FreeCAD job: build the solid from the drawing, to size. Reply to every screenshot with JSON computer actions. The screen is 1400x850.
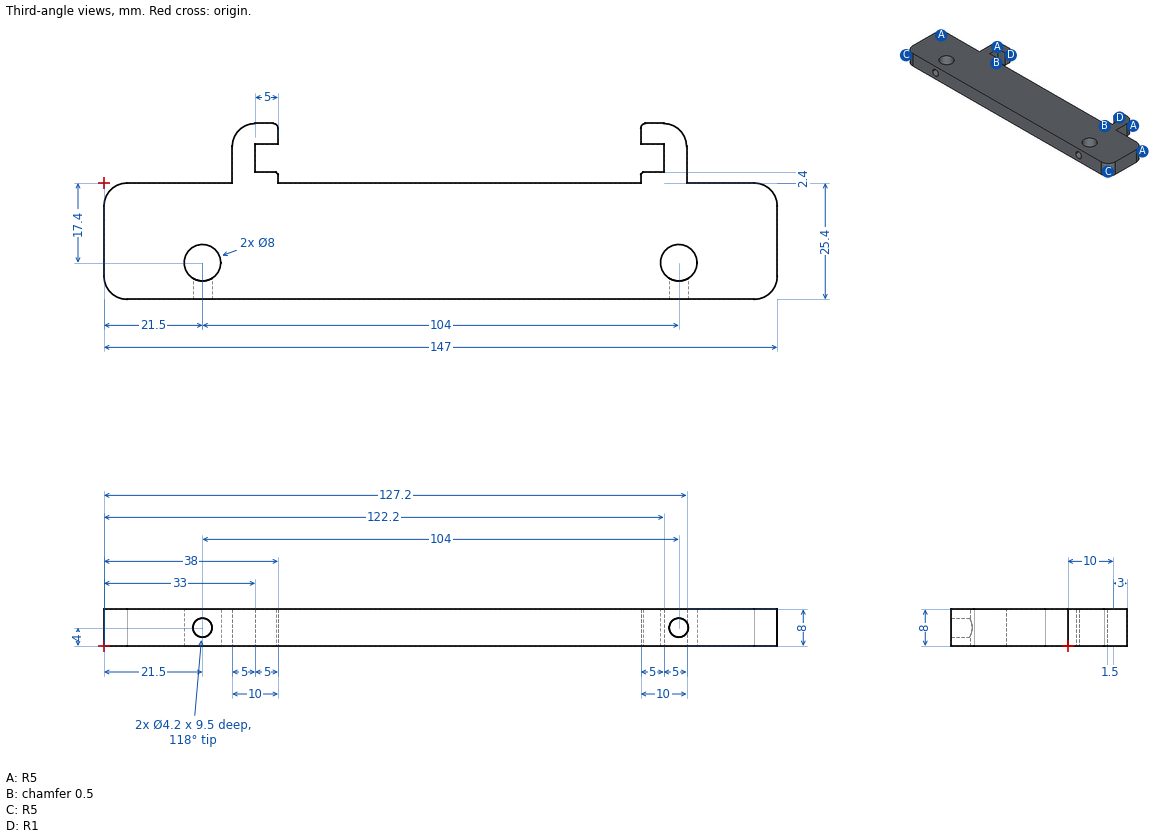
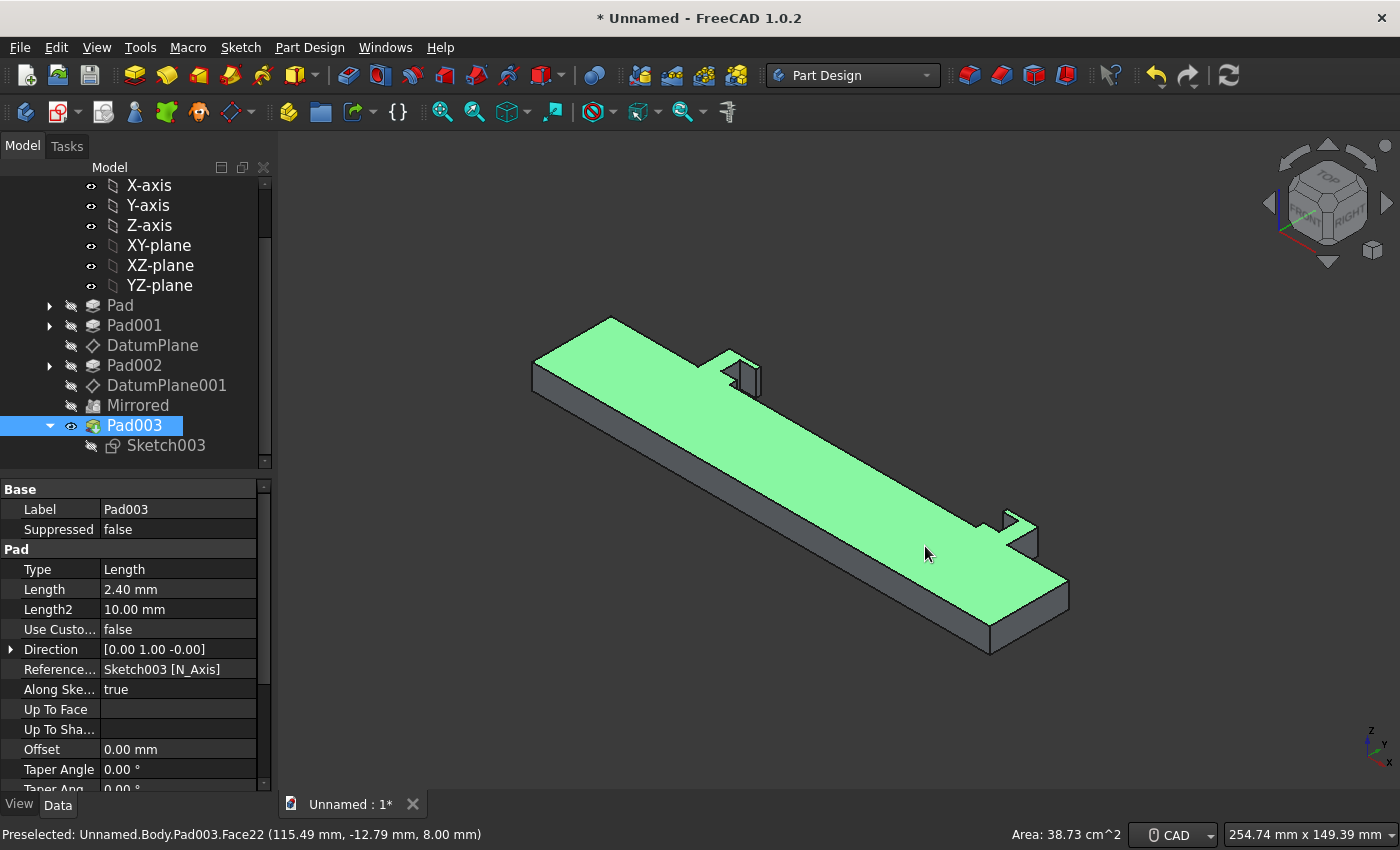
{"action": "left_click", "coordinate": [58, 112]}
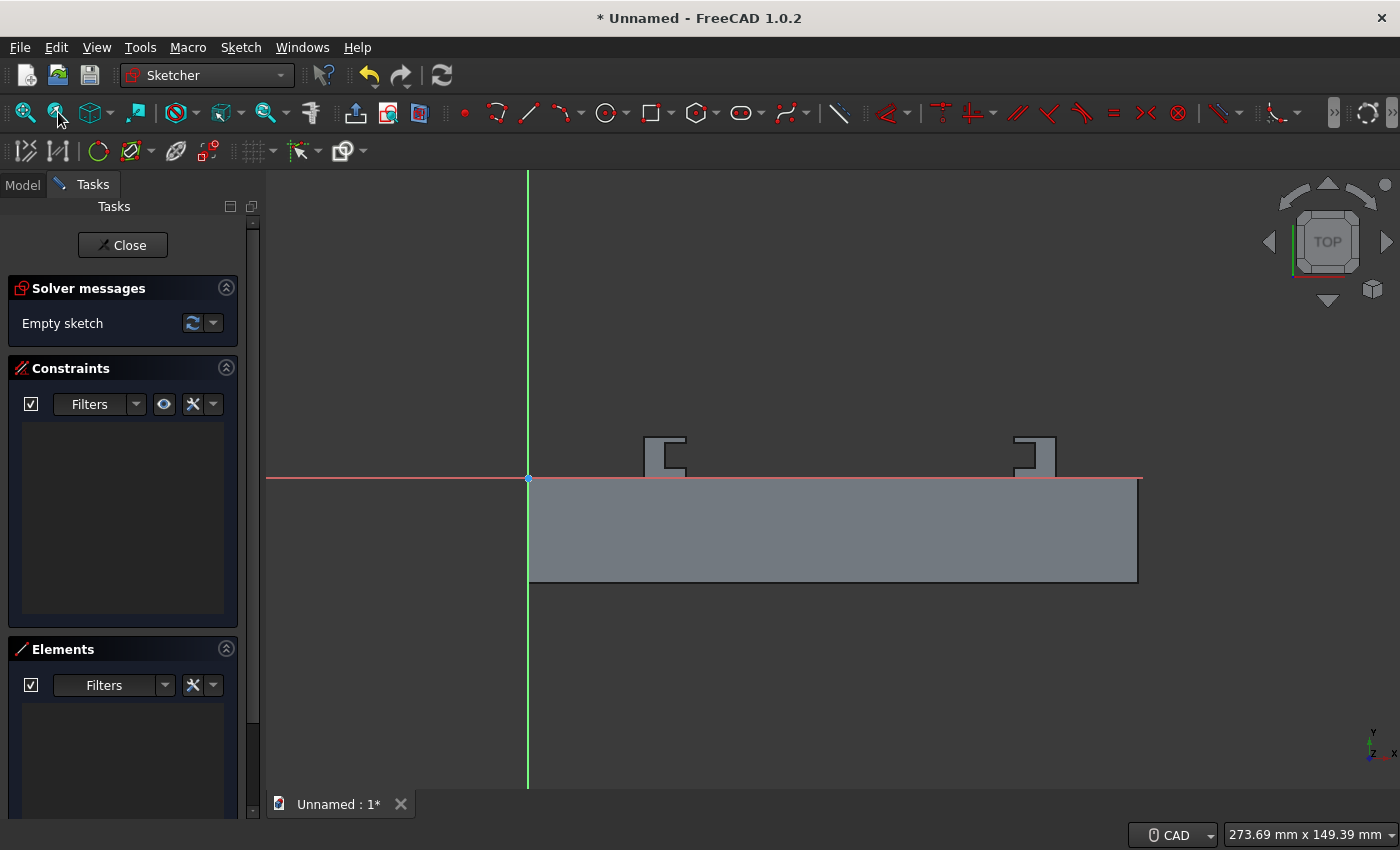
{"action": "left_click", "coordinate": [606, 114]}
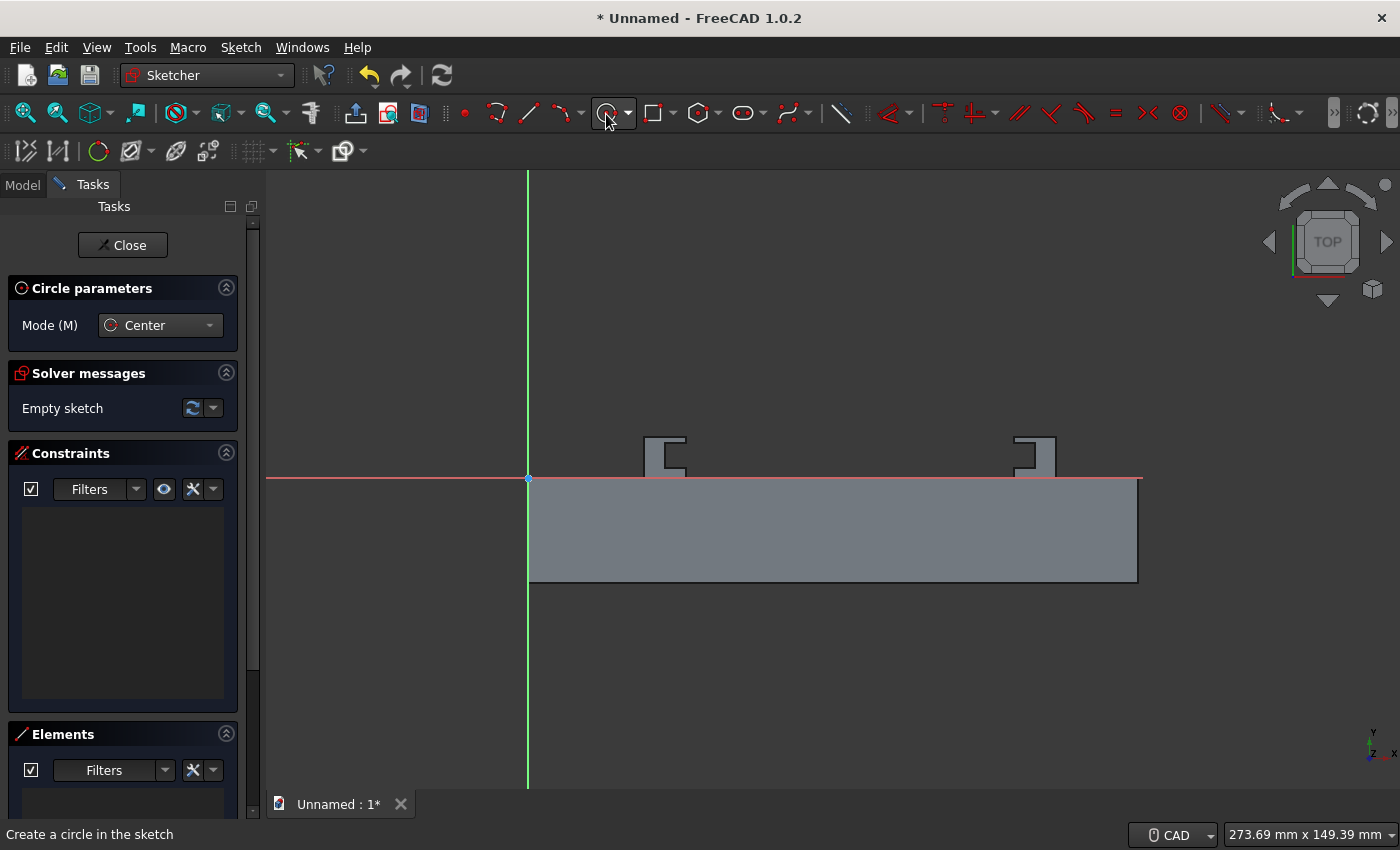
{"action": "scroll", "coordinate": [618, 550], "scroll_direction": "up", "scroll_amount": 2}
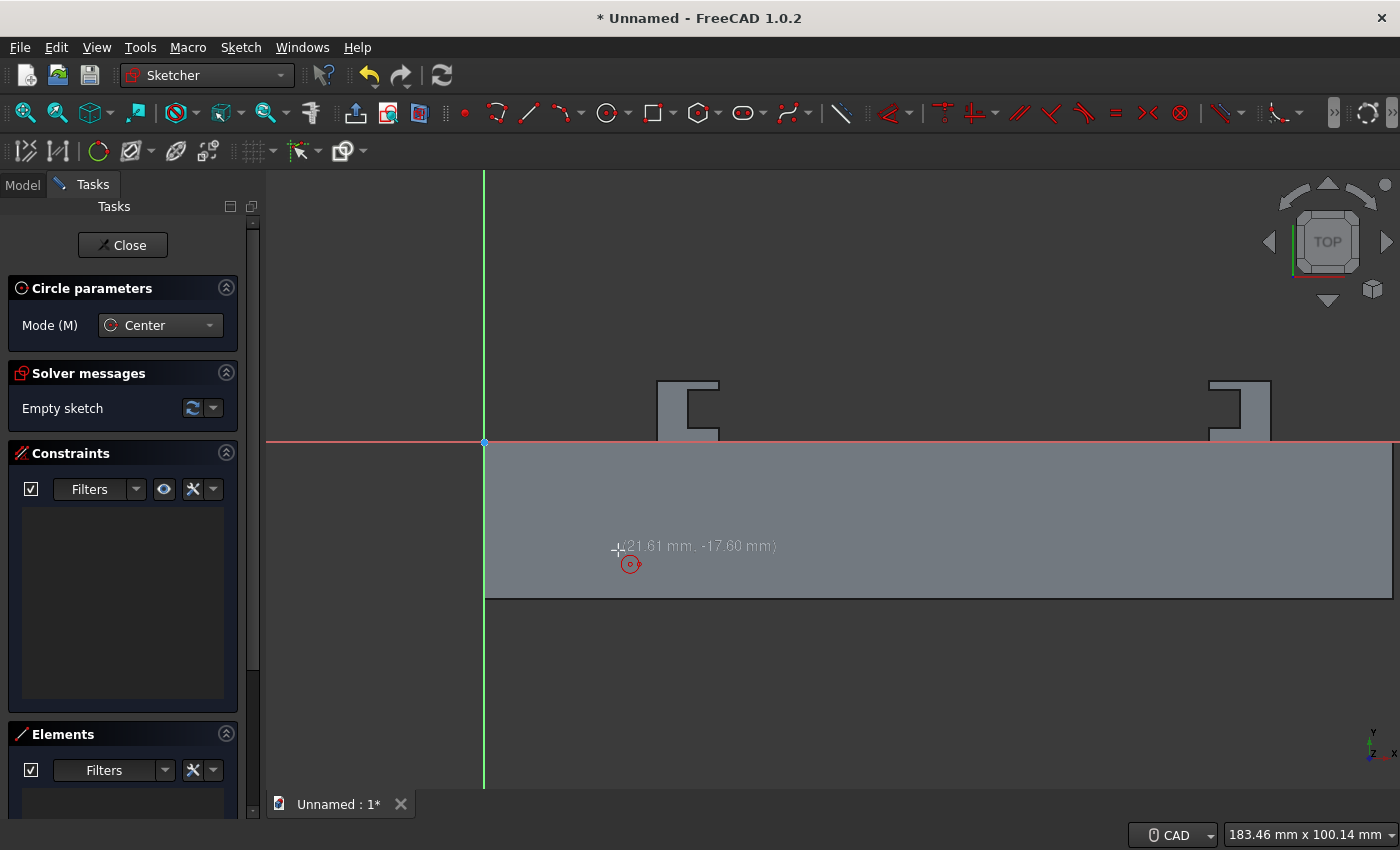
{"action": "left_click", "coordinate": [617, 550]}
{"action": "mouse_move", "coordinate": [635, 532]}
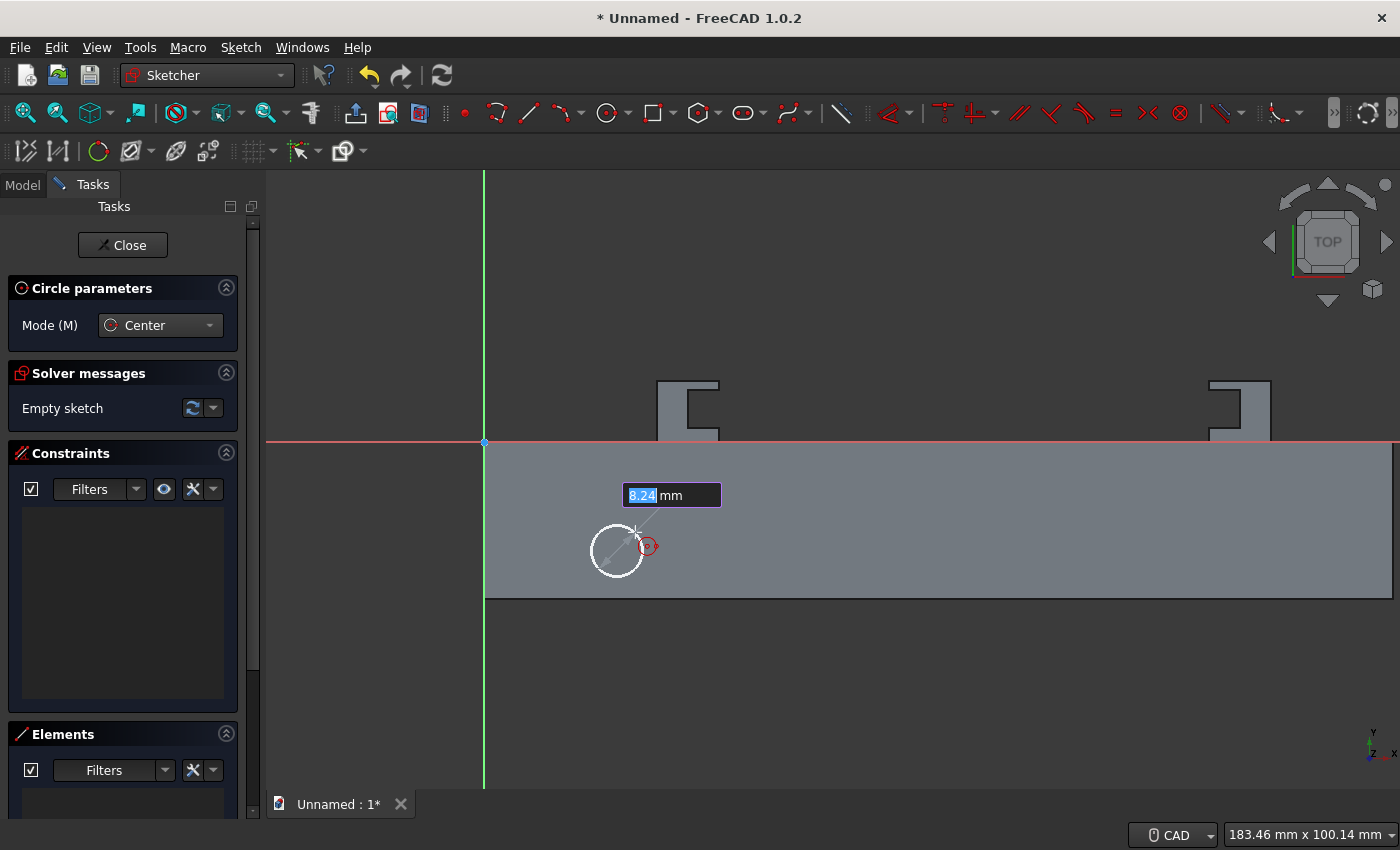
{"action": "type", "text": "8"}
{"action": "key", "text": "Return"}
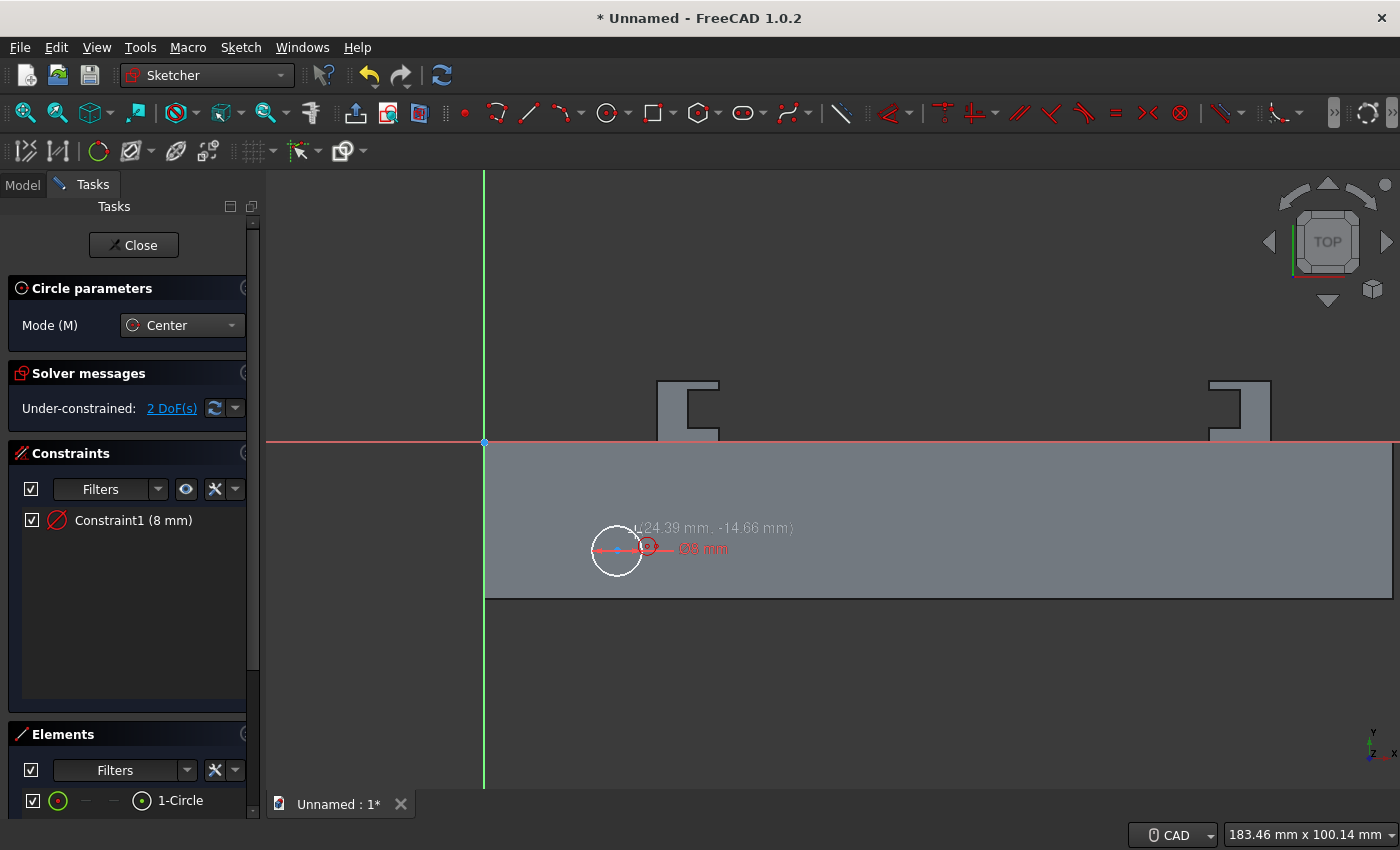
{"action": "scroll", "coordinate": [294, 348], "scroll_direction": "down", "scroll_amount": 1}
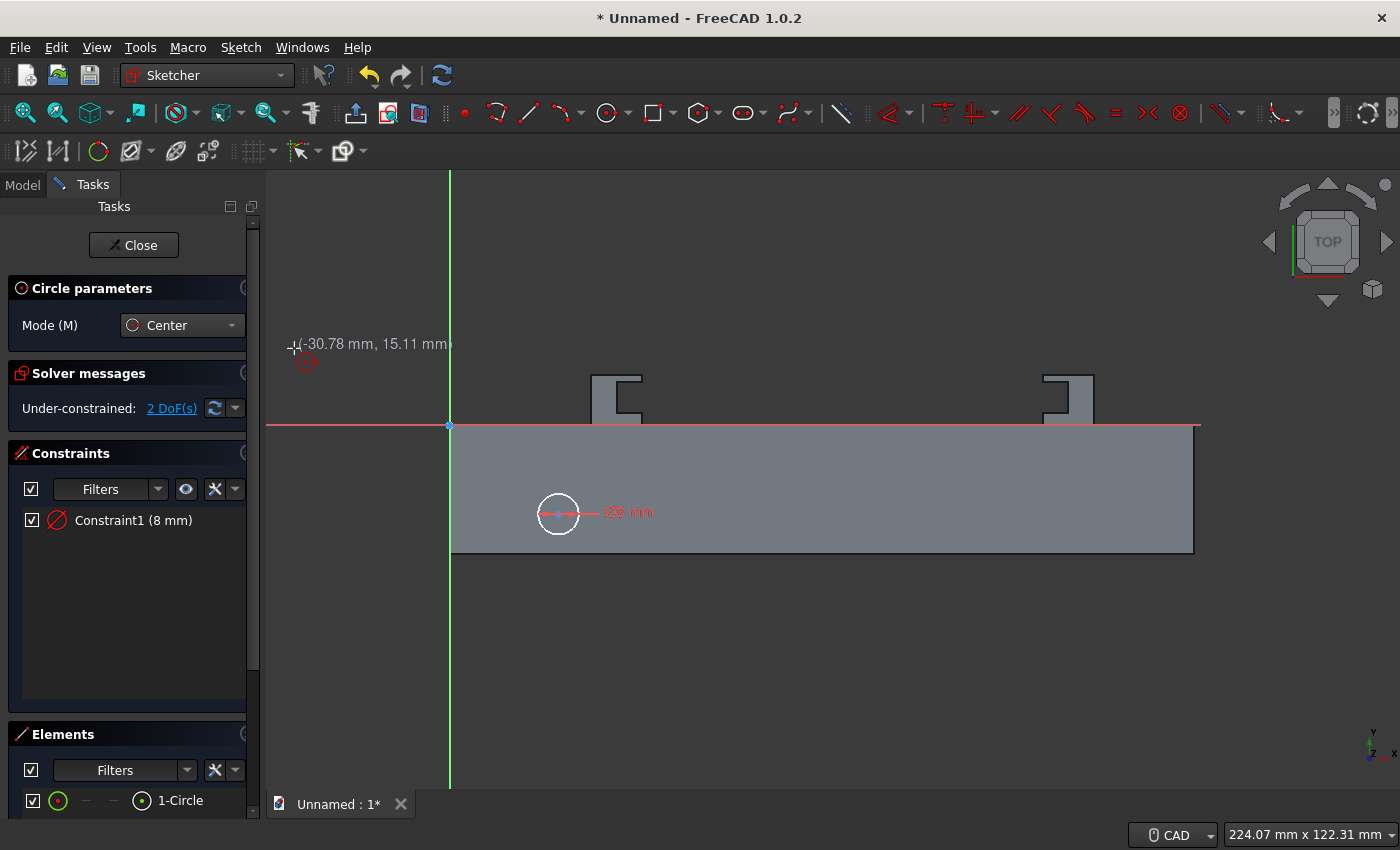
{"action": "left_click", "coordinate": [1085, 513]}
{"action": "mouse_move", "coordinate": [1099, 499]}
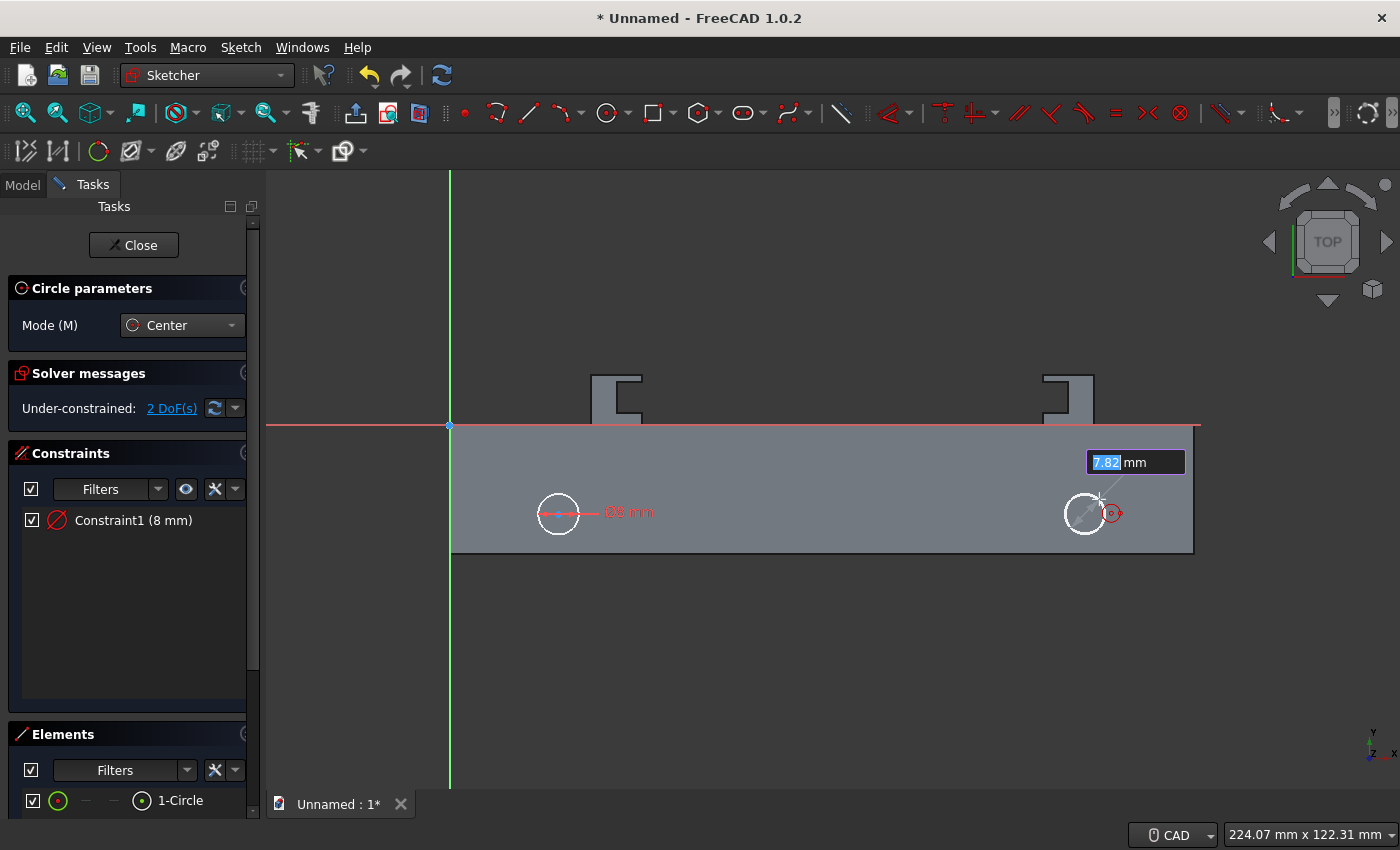
{"action": "type", "text": "8"}
{"action": "key", "text": "Return"}
{"action": "key", "text": "Escape"}